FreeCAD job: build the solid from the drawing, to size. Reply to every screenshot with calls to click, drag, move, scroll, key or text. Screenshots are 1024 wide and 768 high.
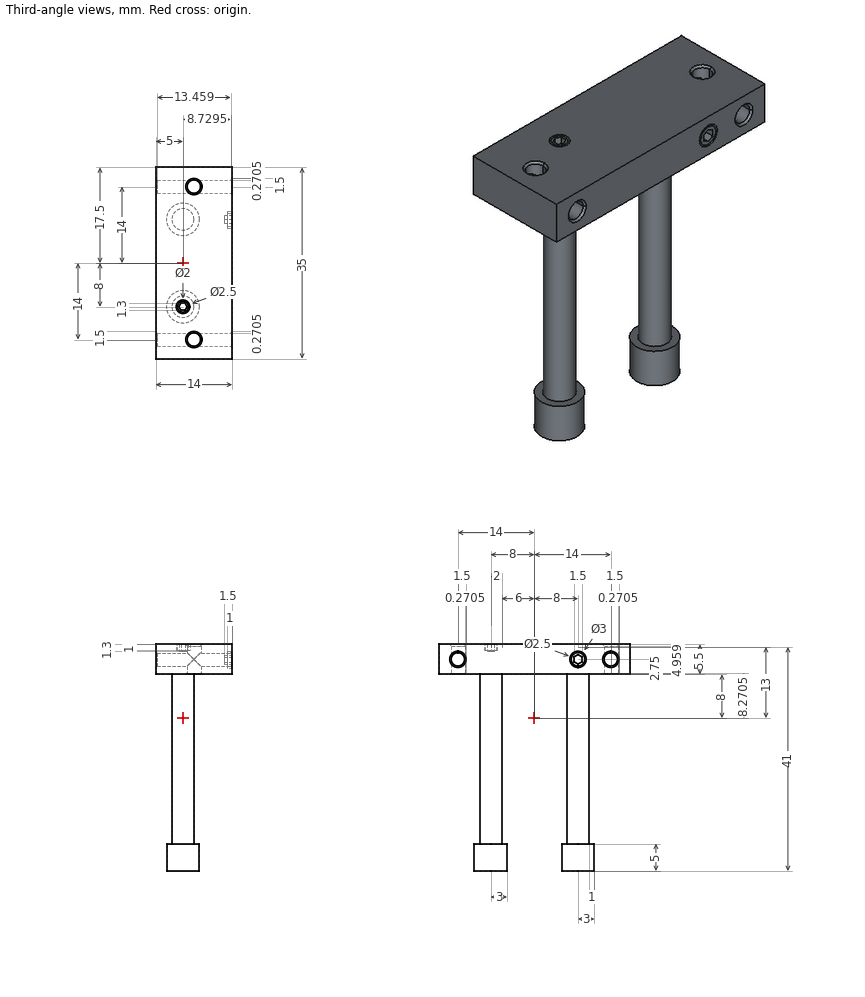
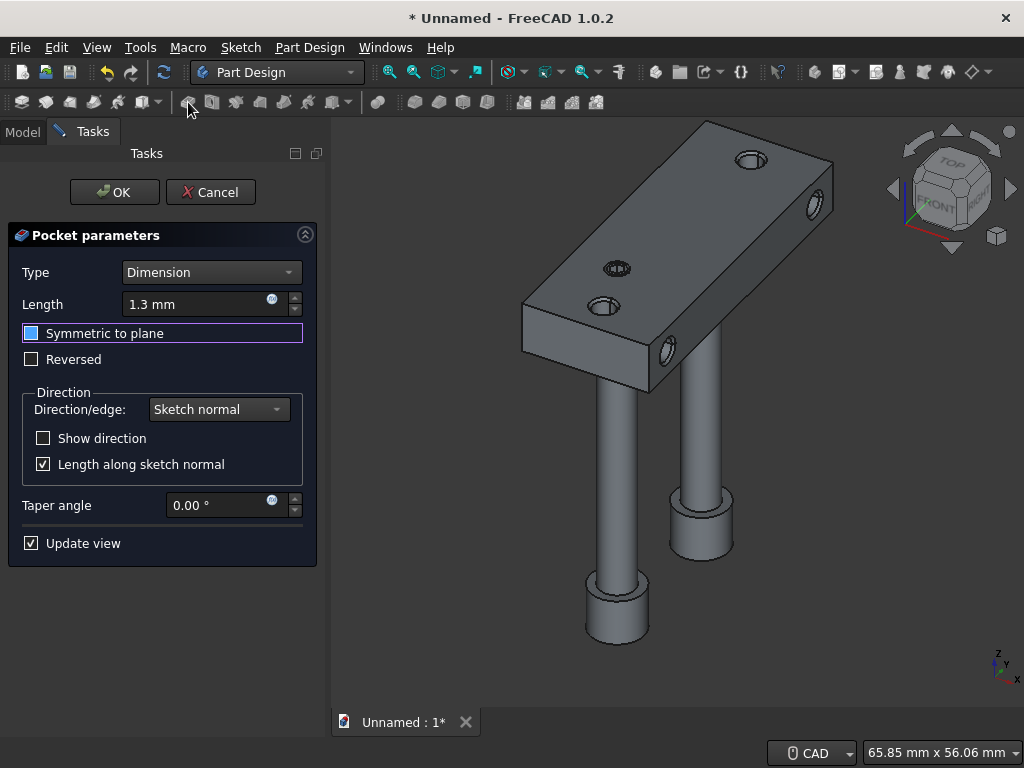
click(115, 192)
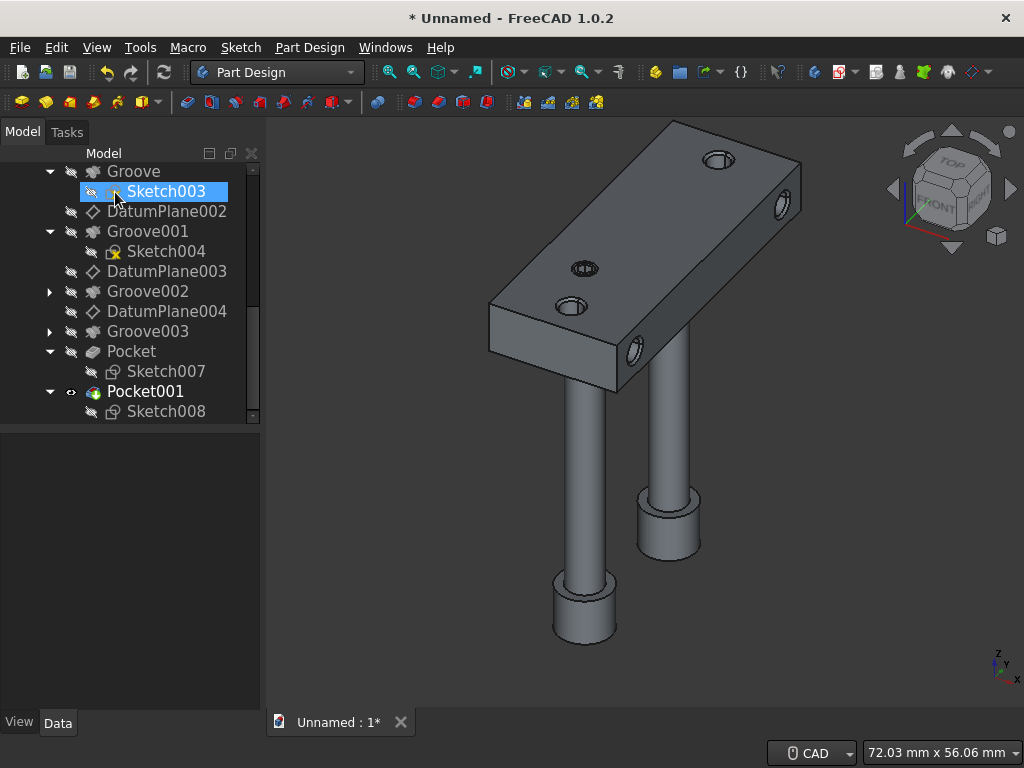
click(735, 251)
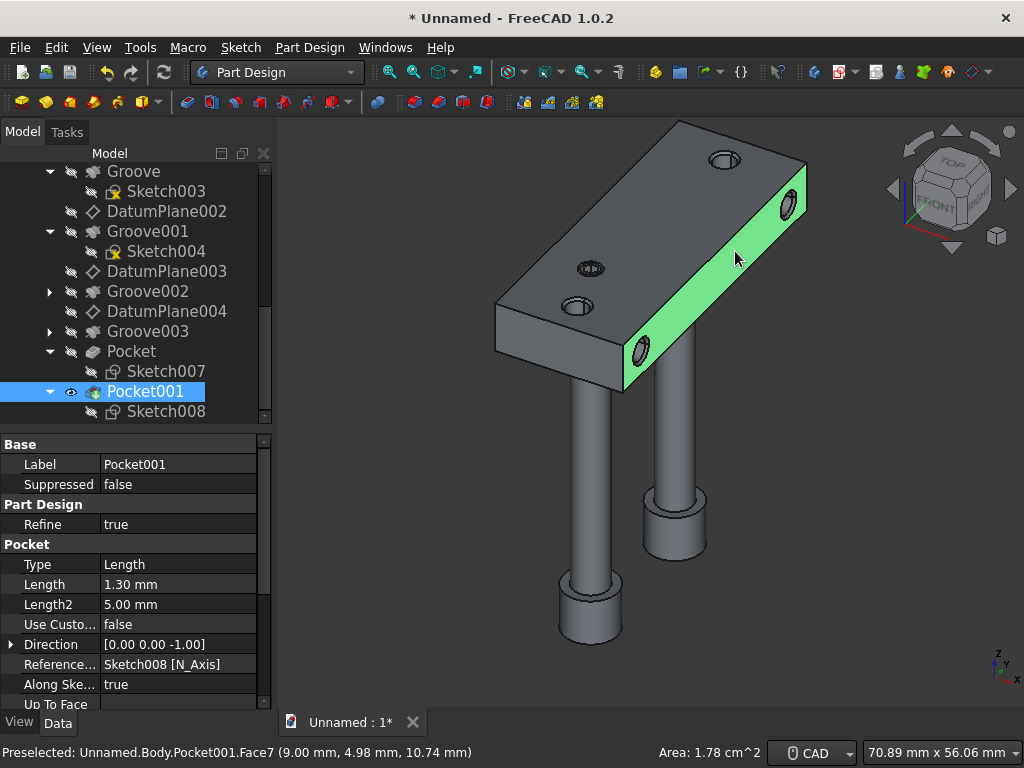
click(840, 72)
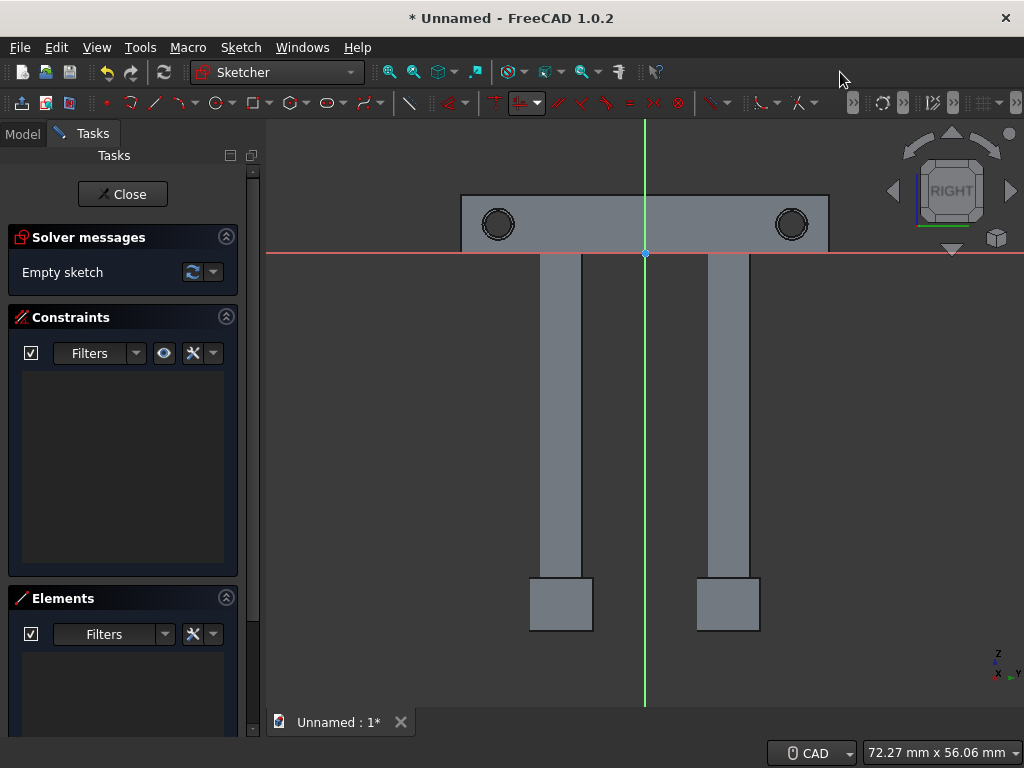
scroll(744, 205, up, 12)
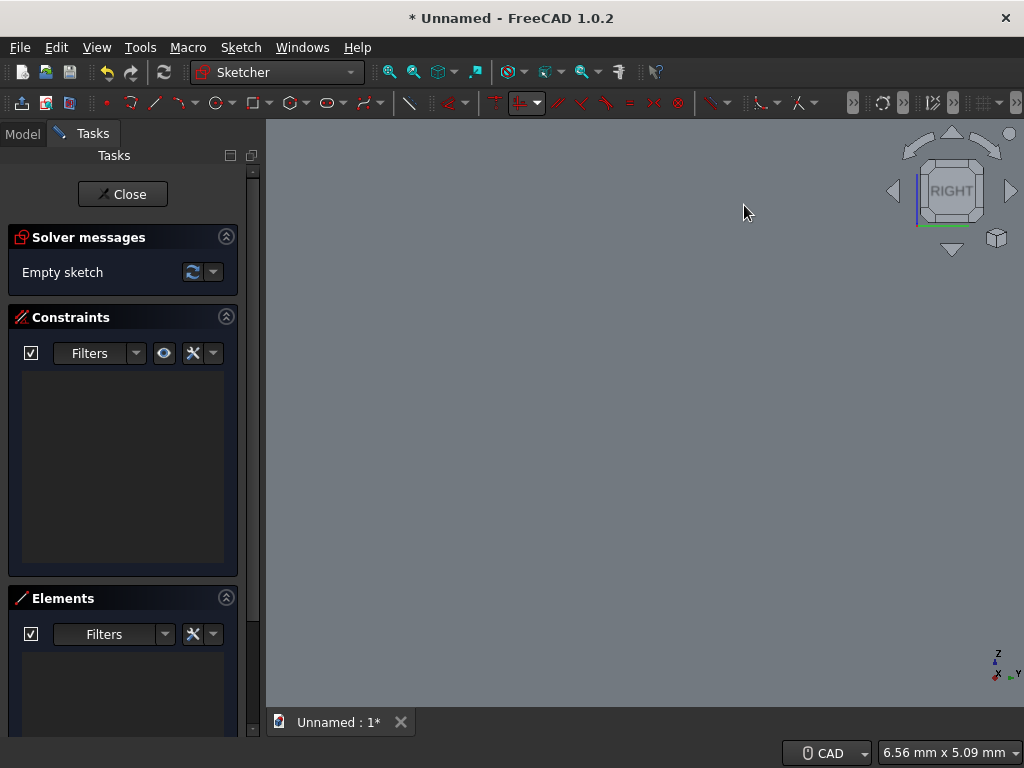
click(216, 104)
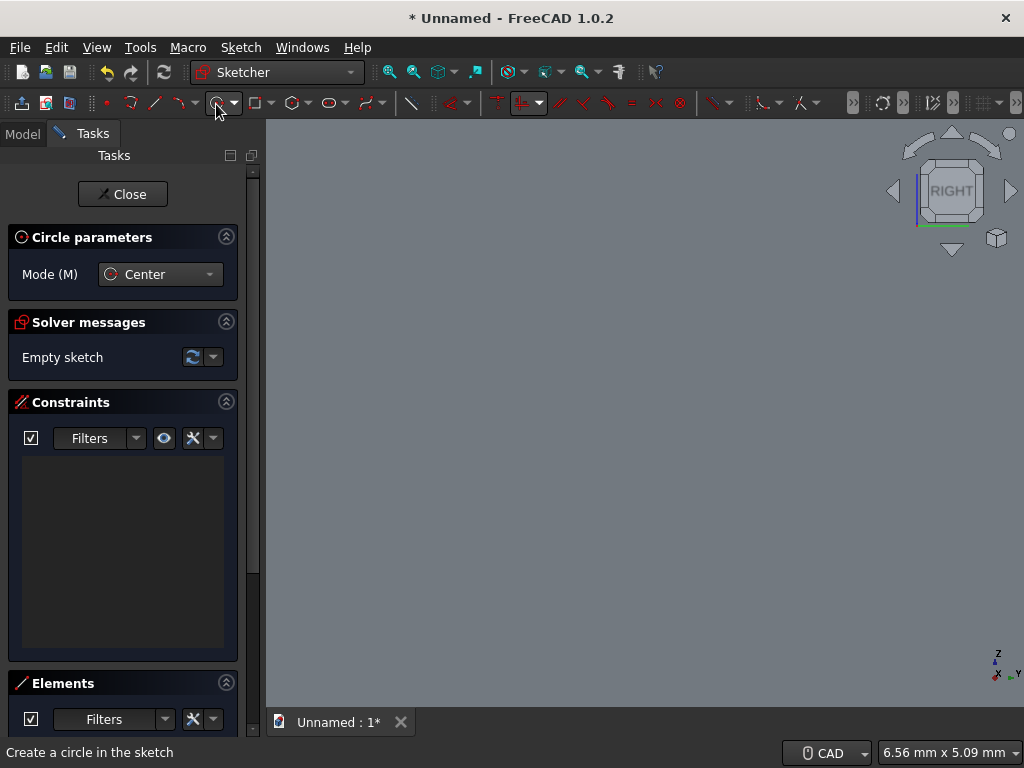
click(571, 415)
move(694, 293)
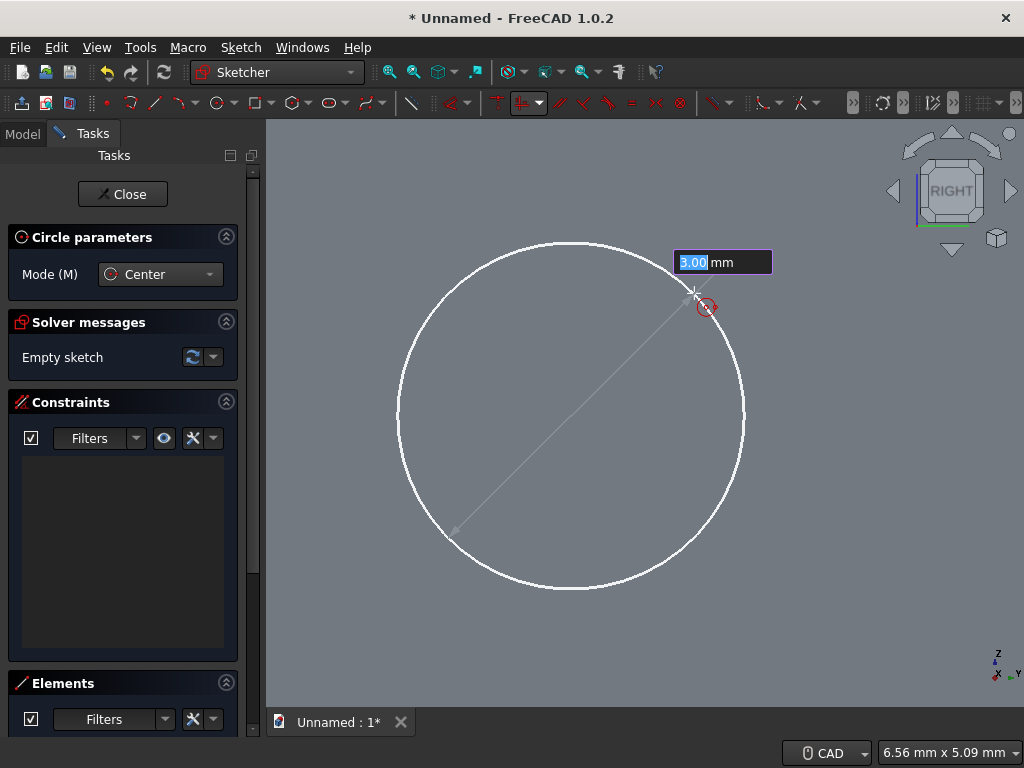
text(3)
key(Return)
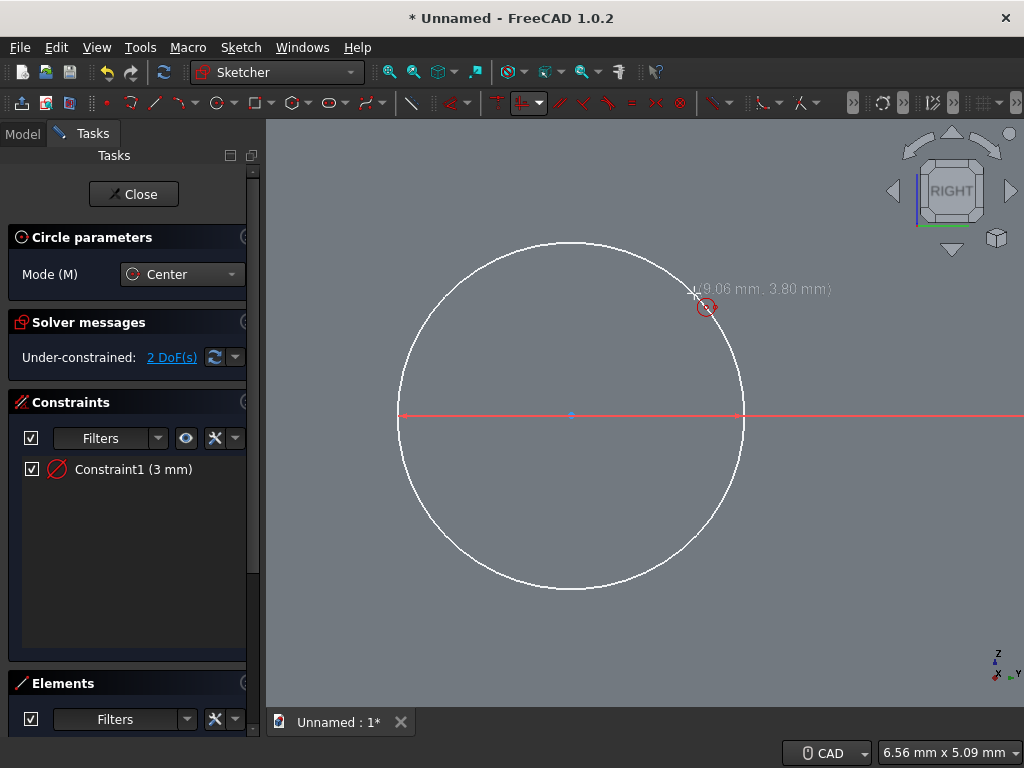
click(571, 416)
move(673, 313)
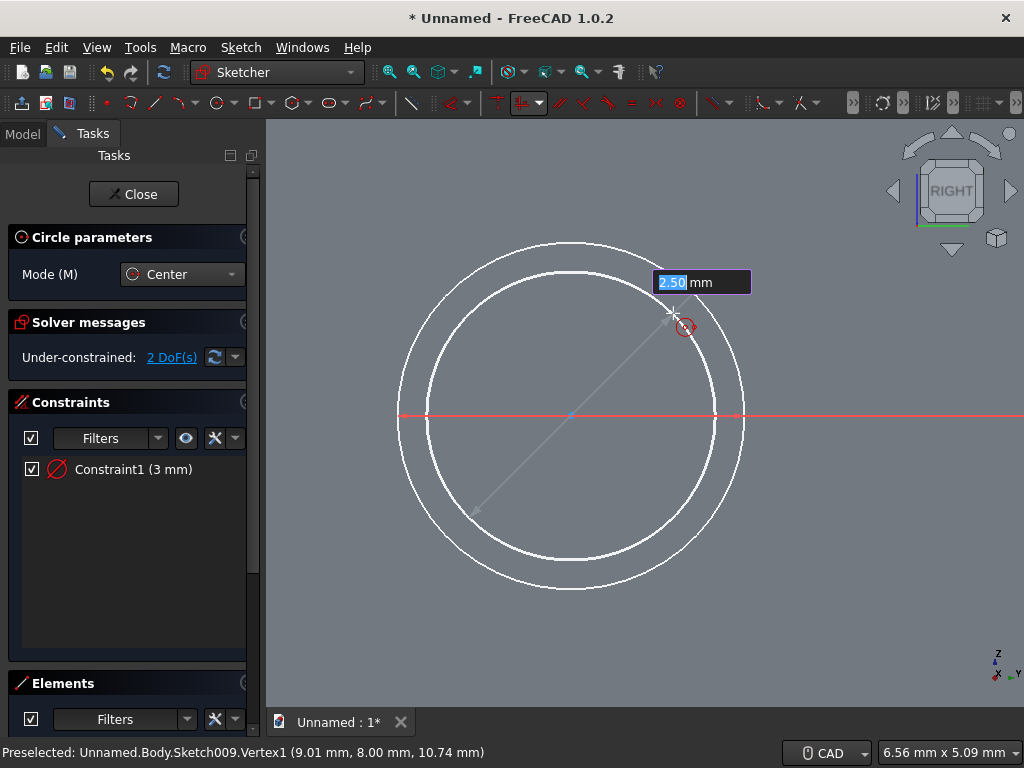
text(2.5)
key(Return)
key(Escape)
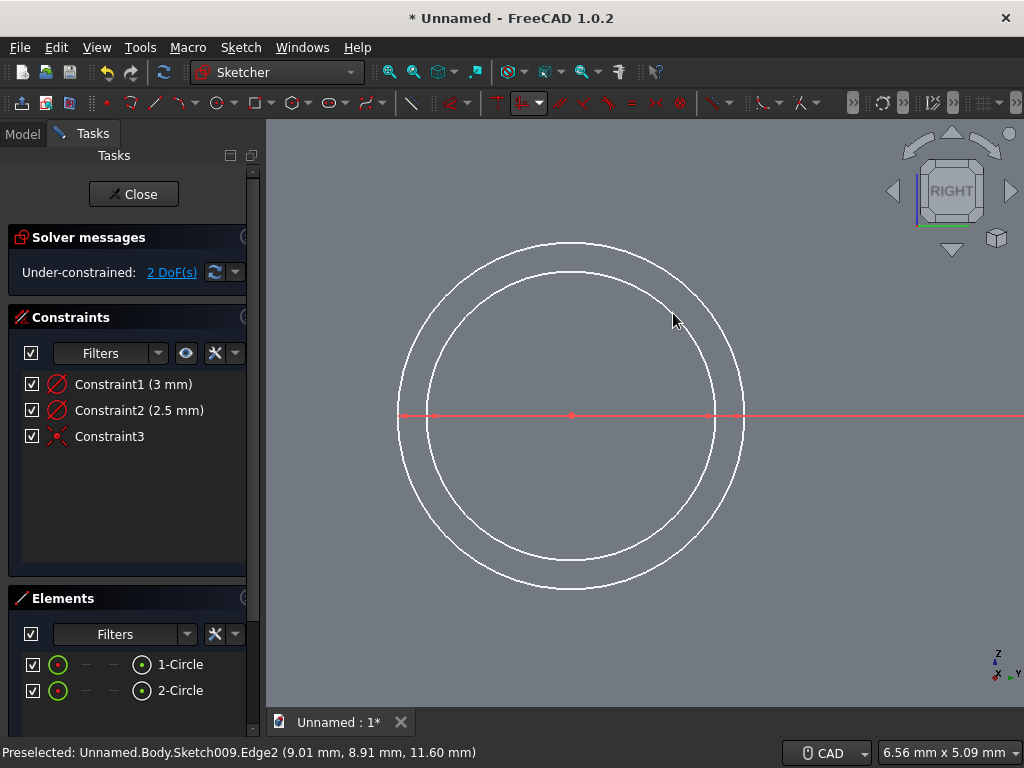
click(450, 104)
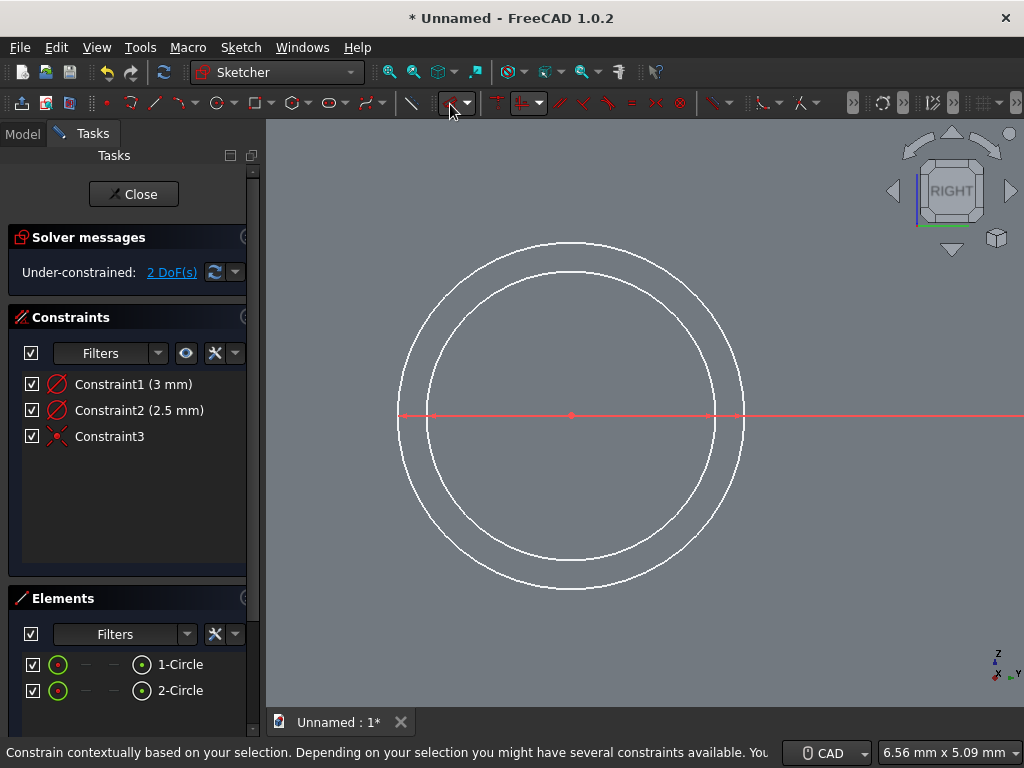
click(571, 416)
click(369, 382)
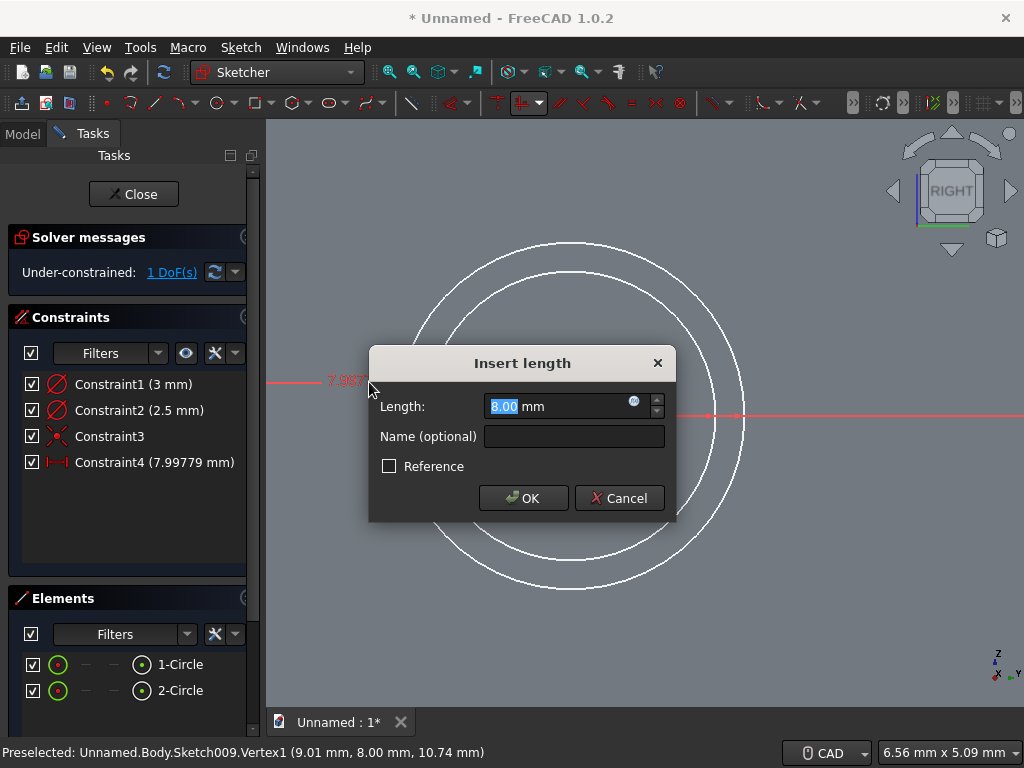
text(8)
key(Return)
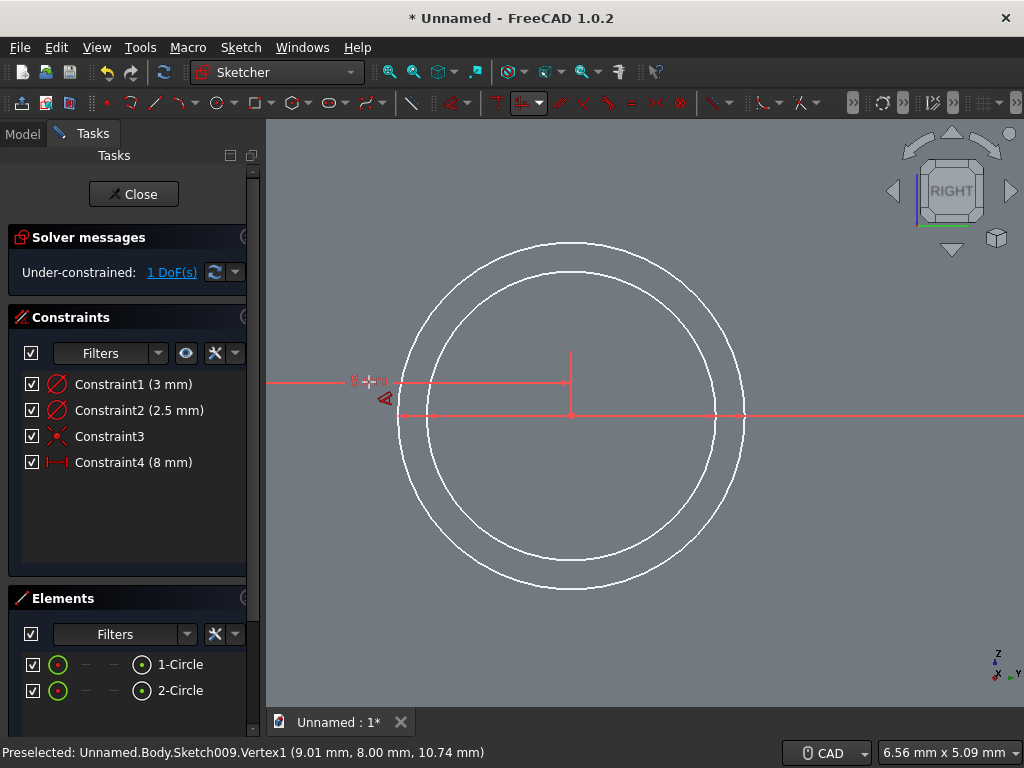
click(571, 416)
click(605, 487)